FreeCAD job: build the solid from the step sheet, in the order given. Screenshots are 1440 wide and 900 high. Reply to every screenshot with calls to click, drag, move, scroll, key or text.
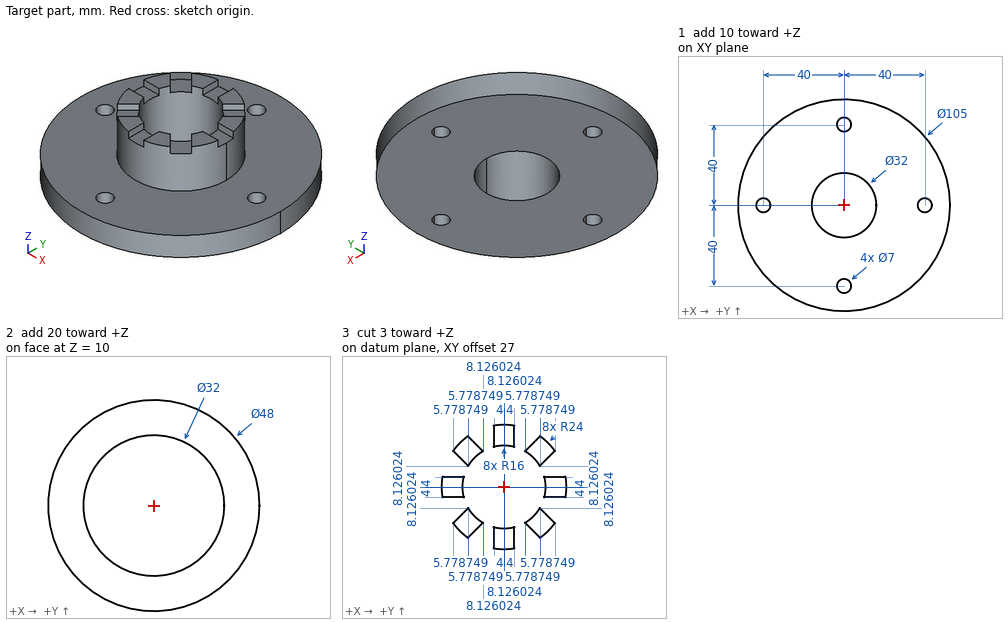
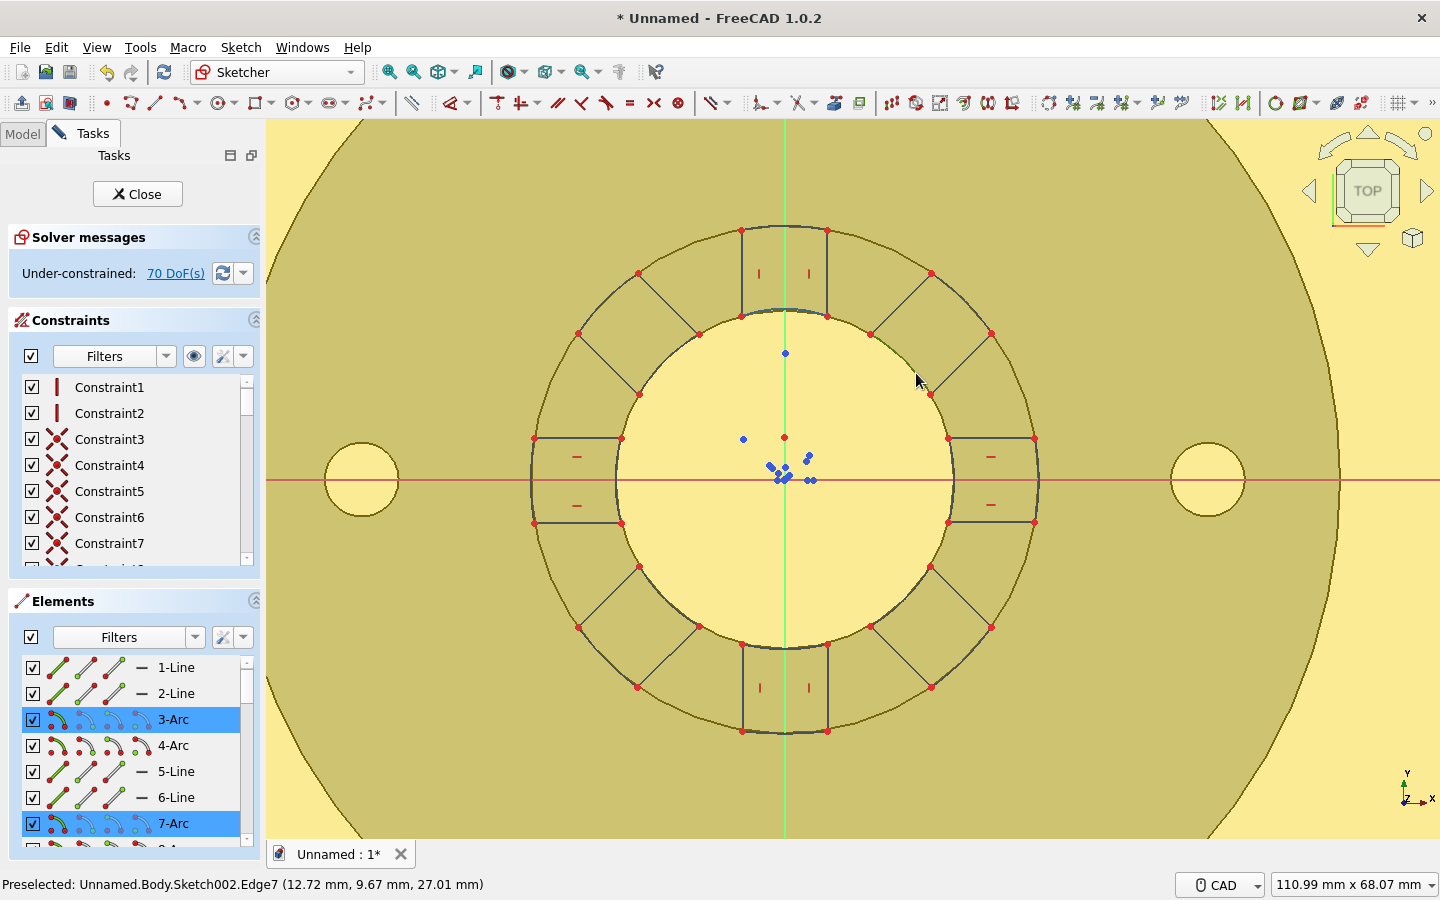
click(498, 104)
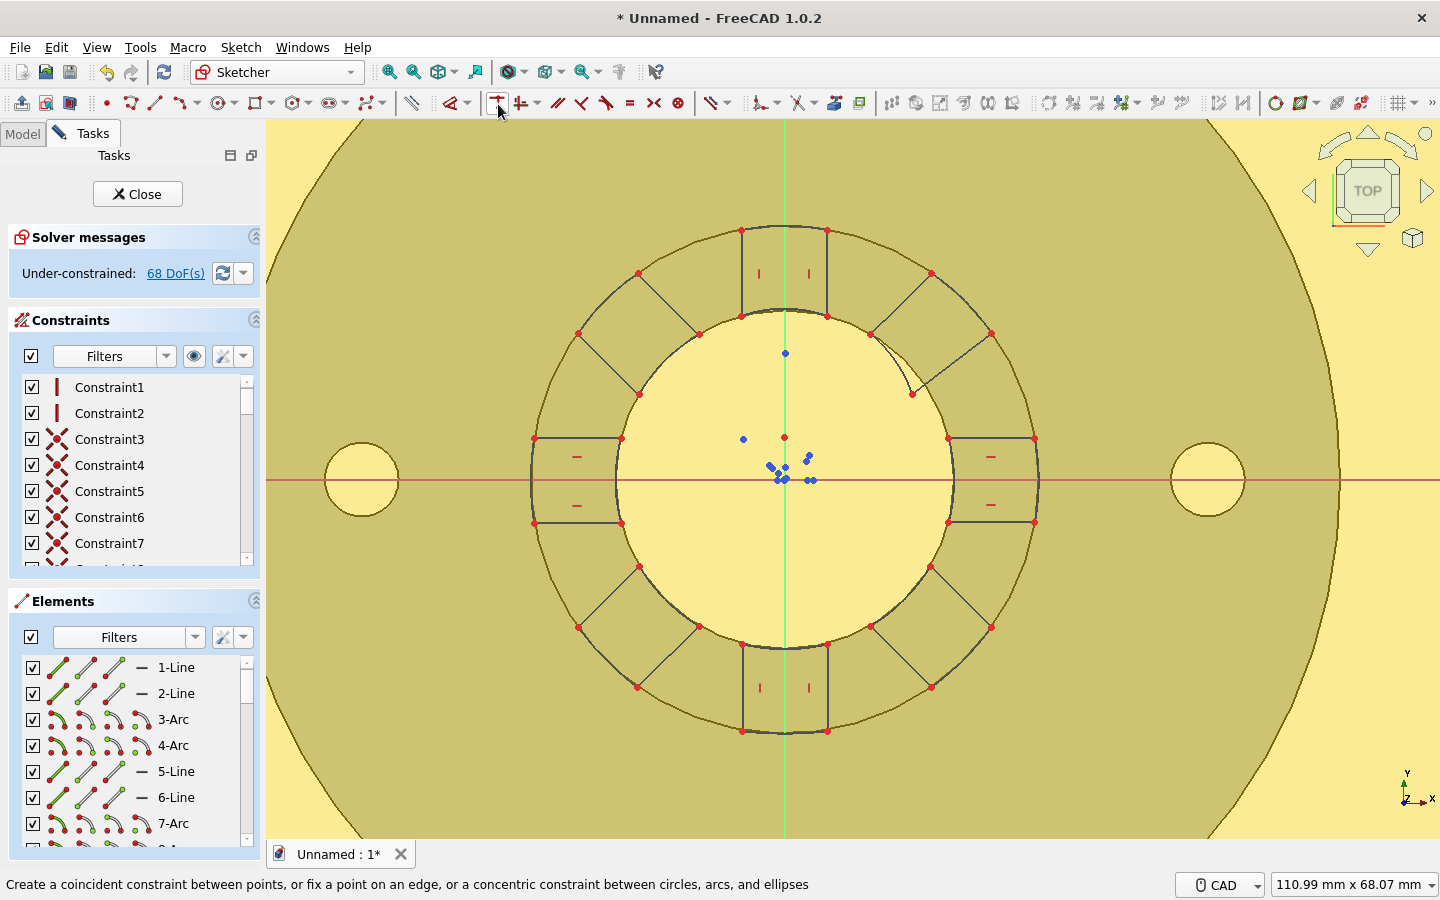
click(802, 310)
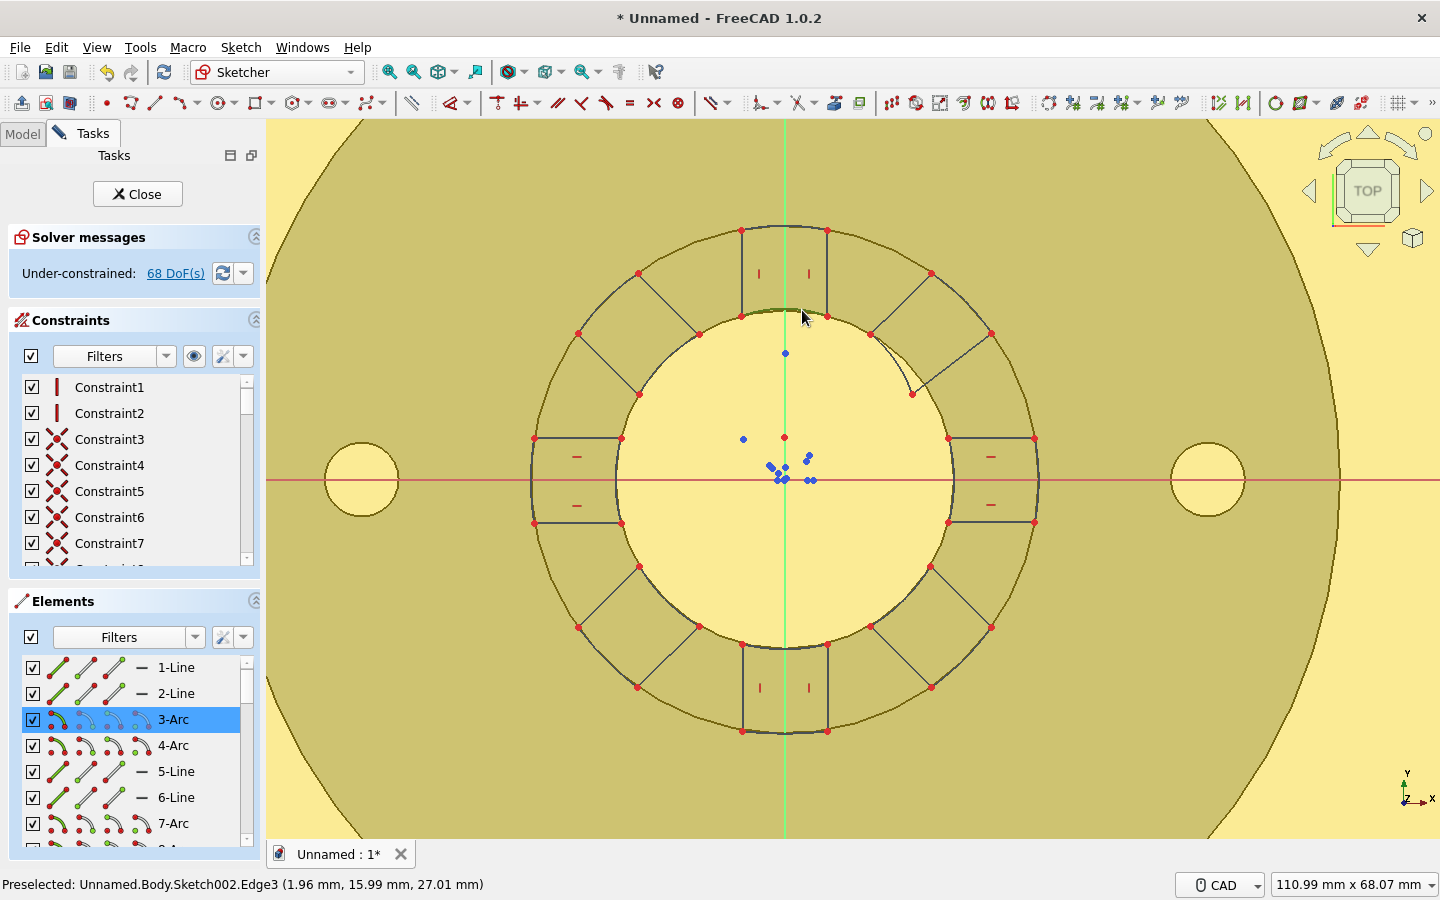
click(976, 313)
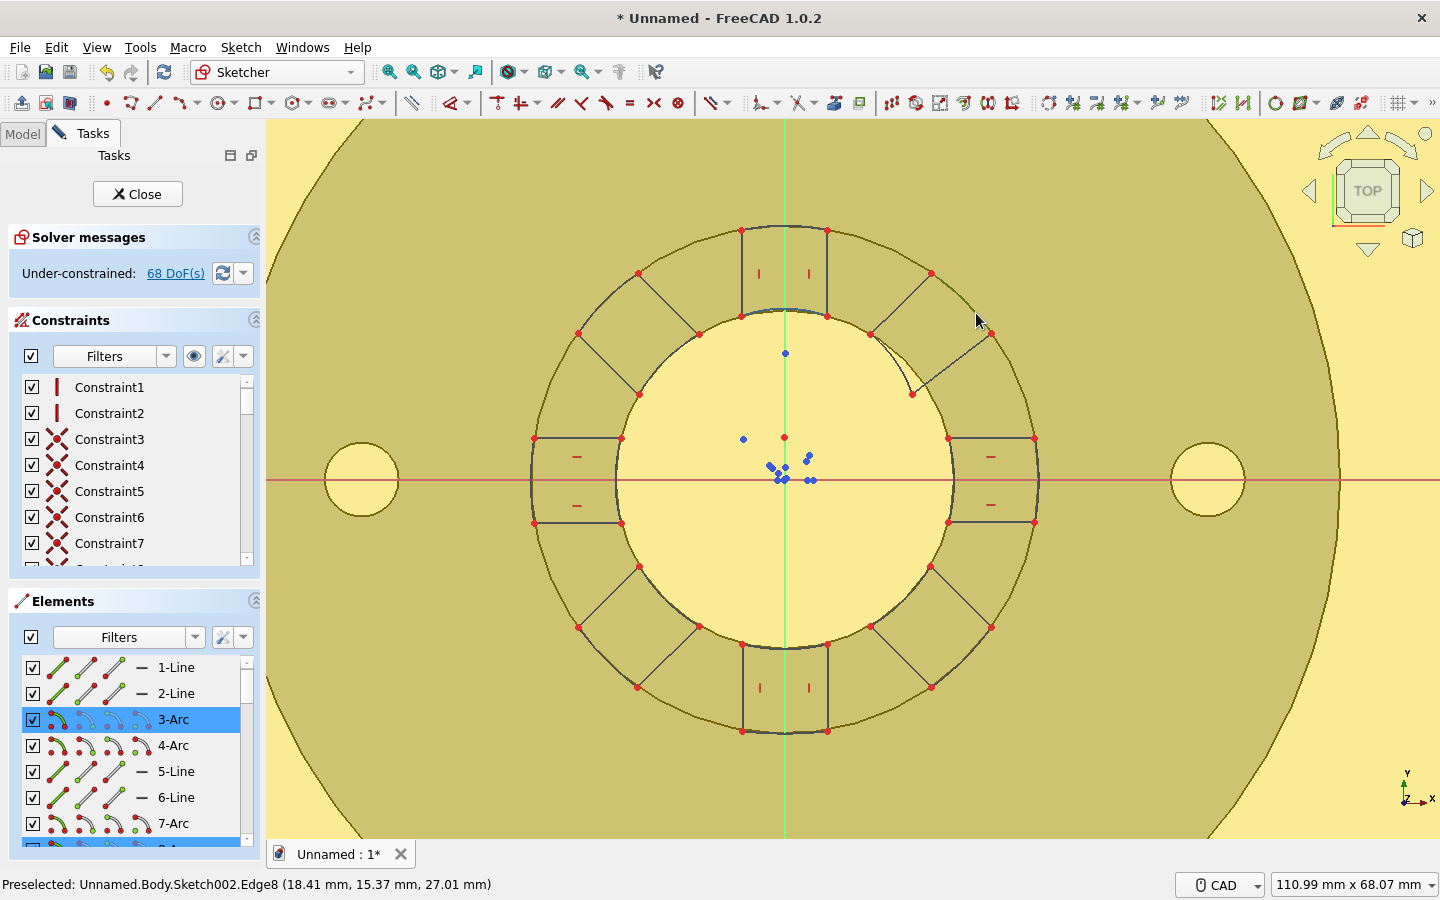
click(498, 104)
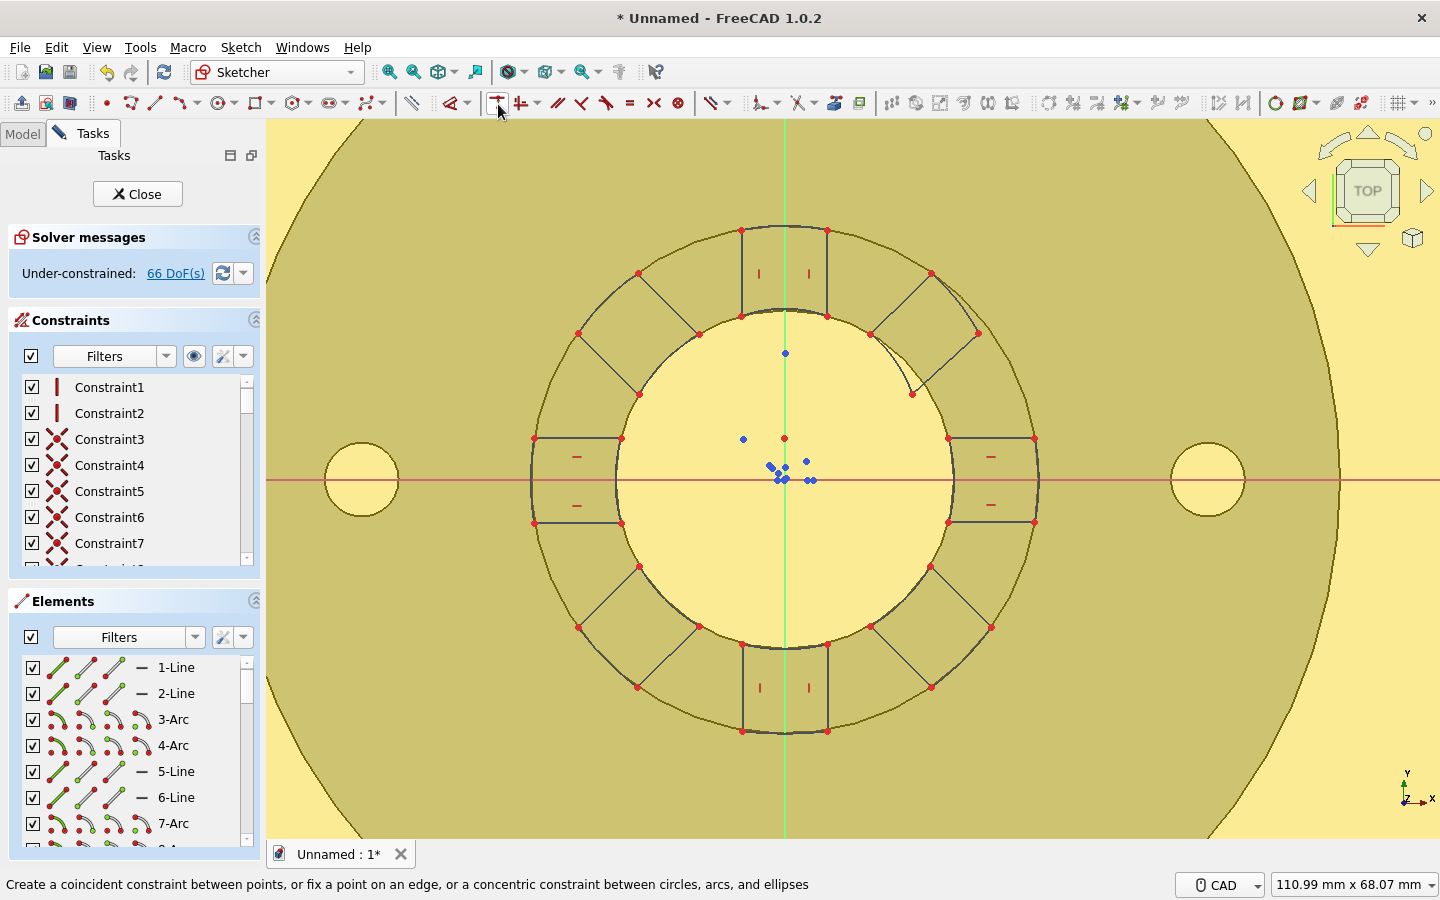
click(802, 310)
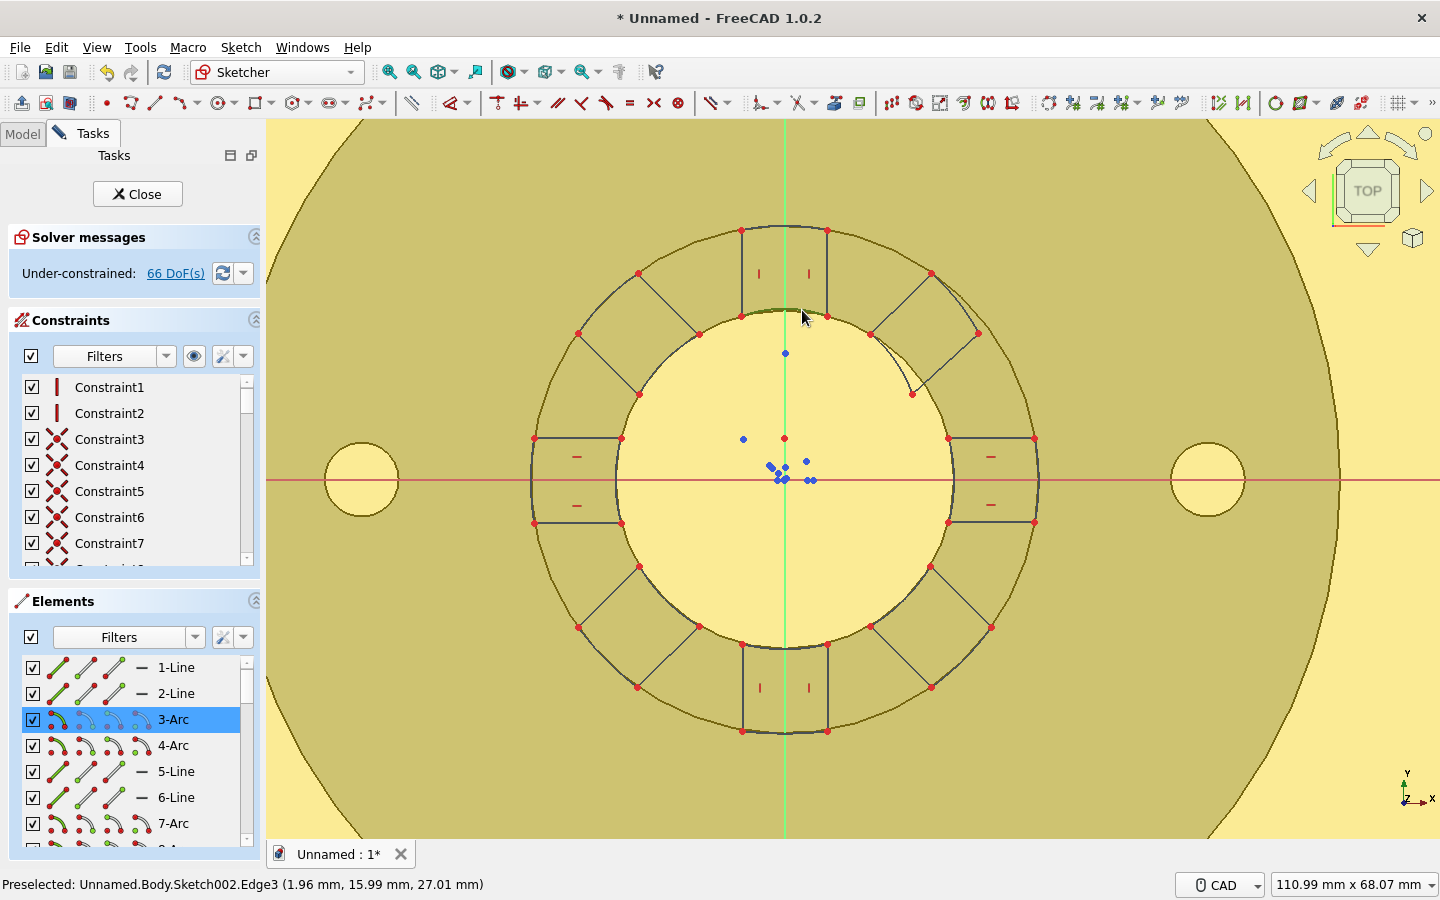
click(953, 497)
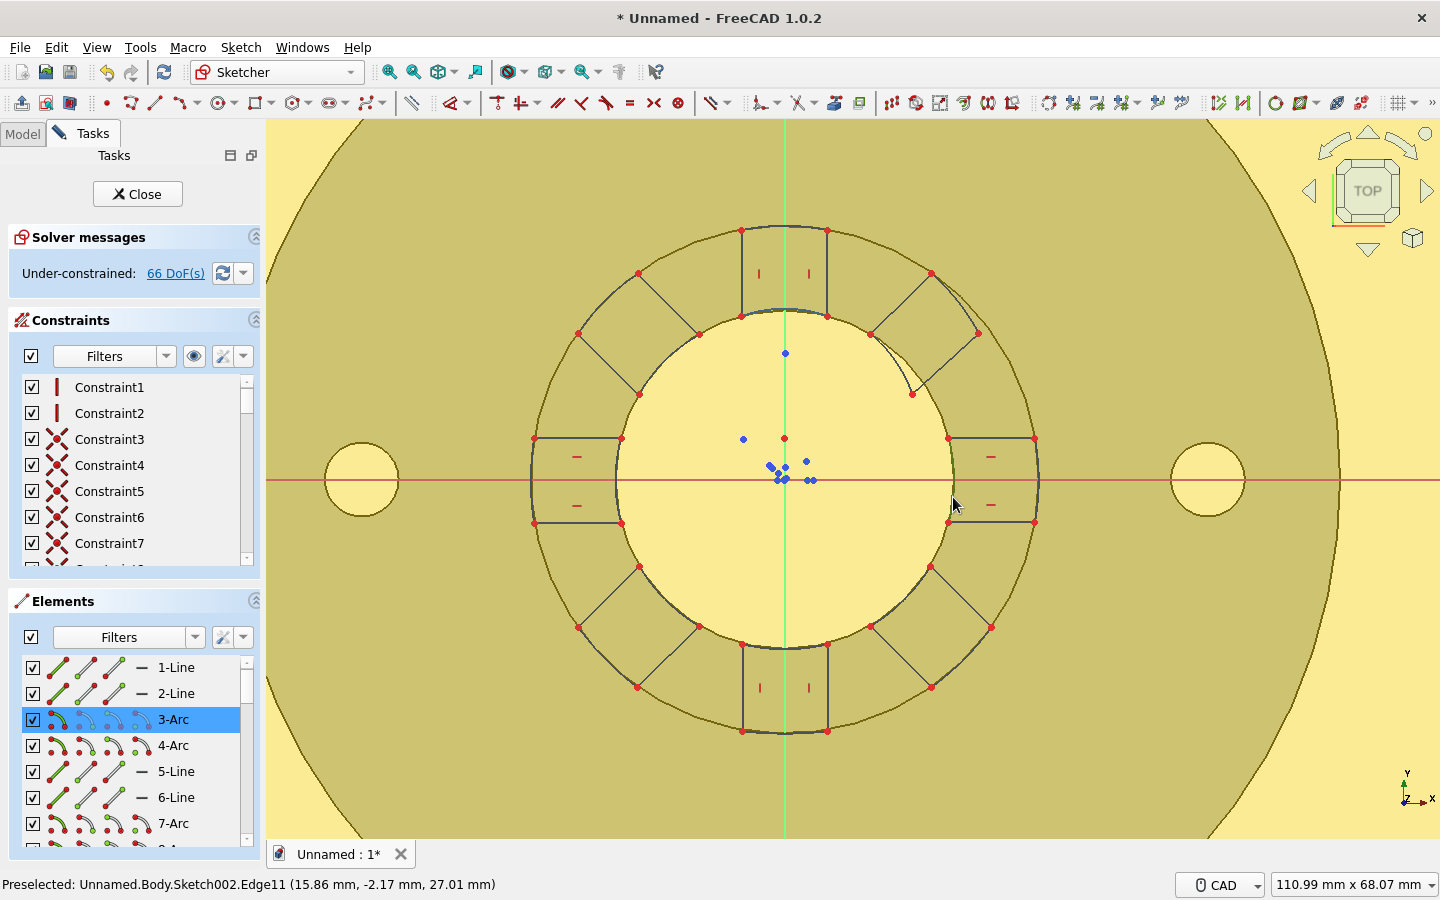
click(498, 104)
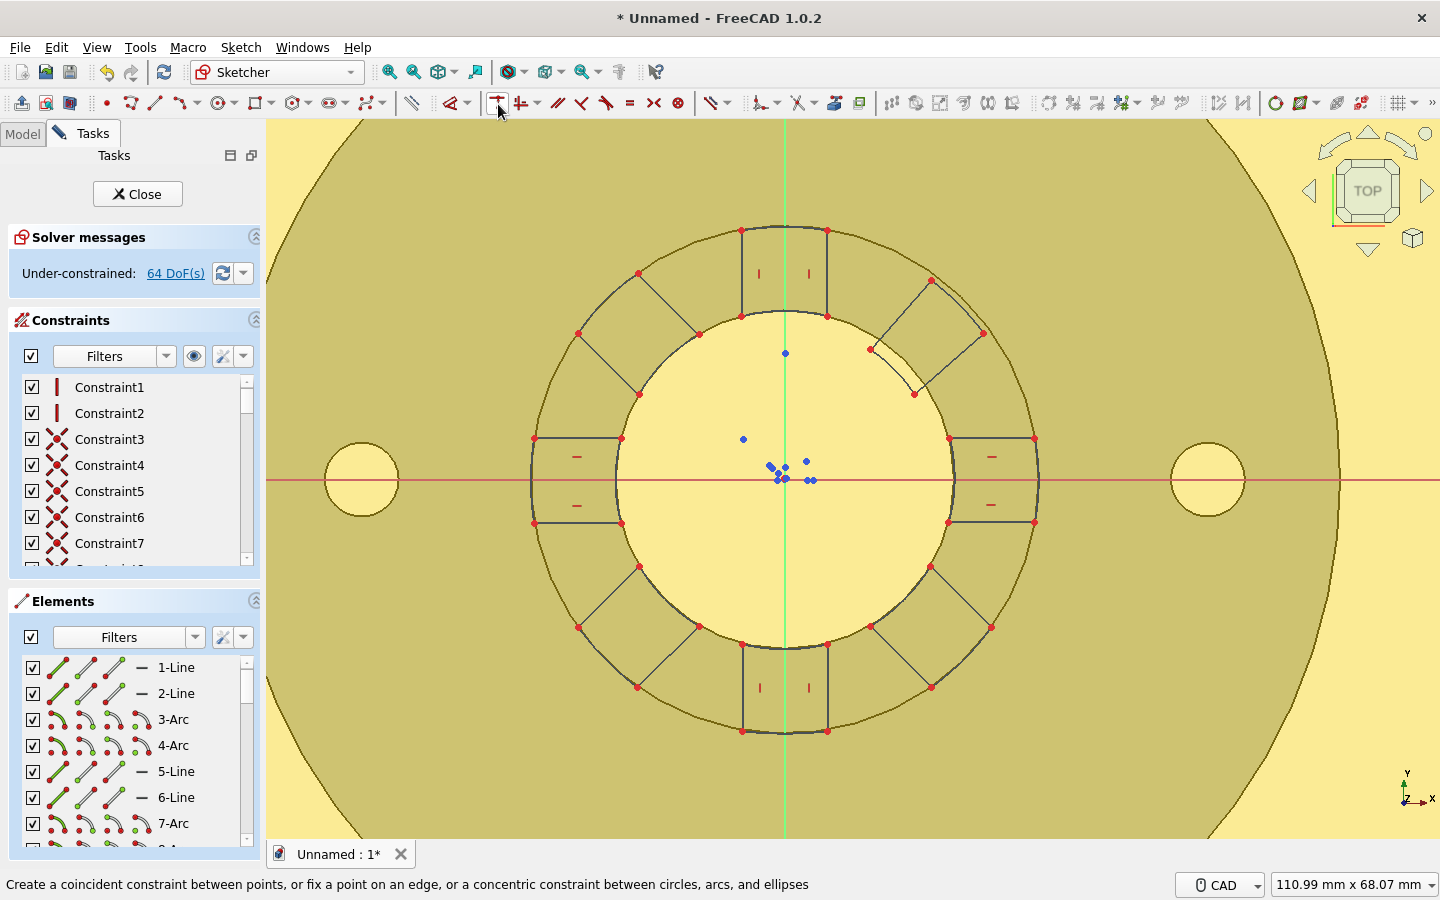
click(802, 312)